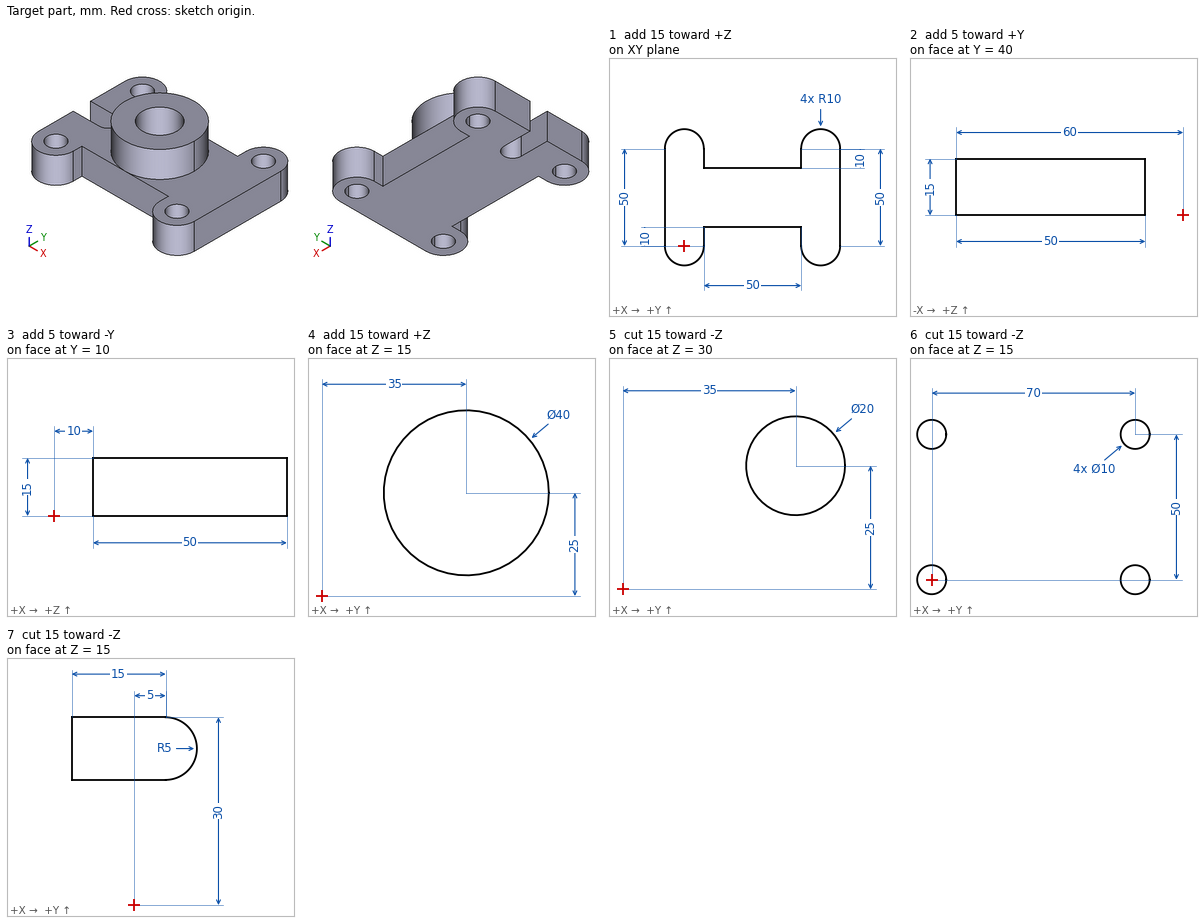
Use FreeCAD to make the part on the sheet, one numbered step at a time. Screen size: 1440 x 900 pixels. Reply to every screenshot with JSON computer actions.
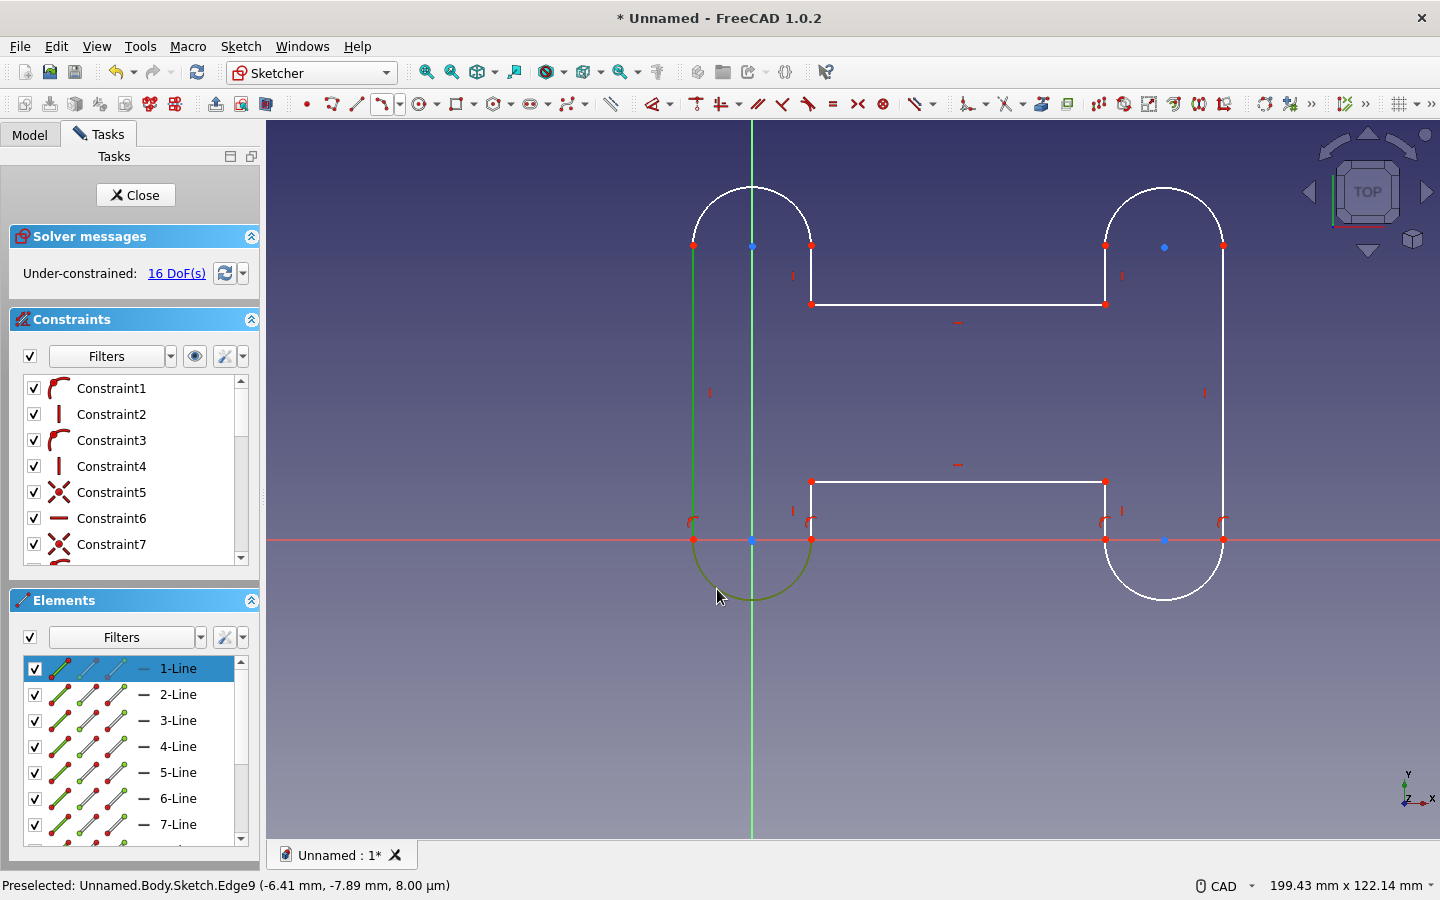
{"action": "key", "text": "t"}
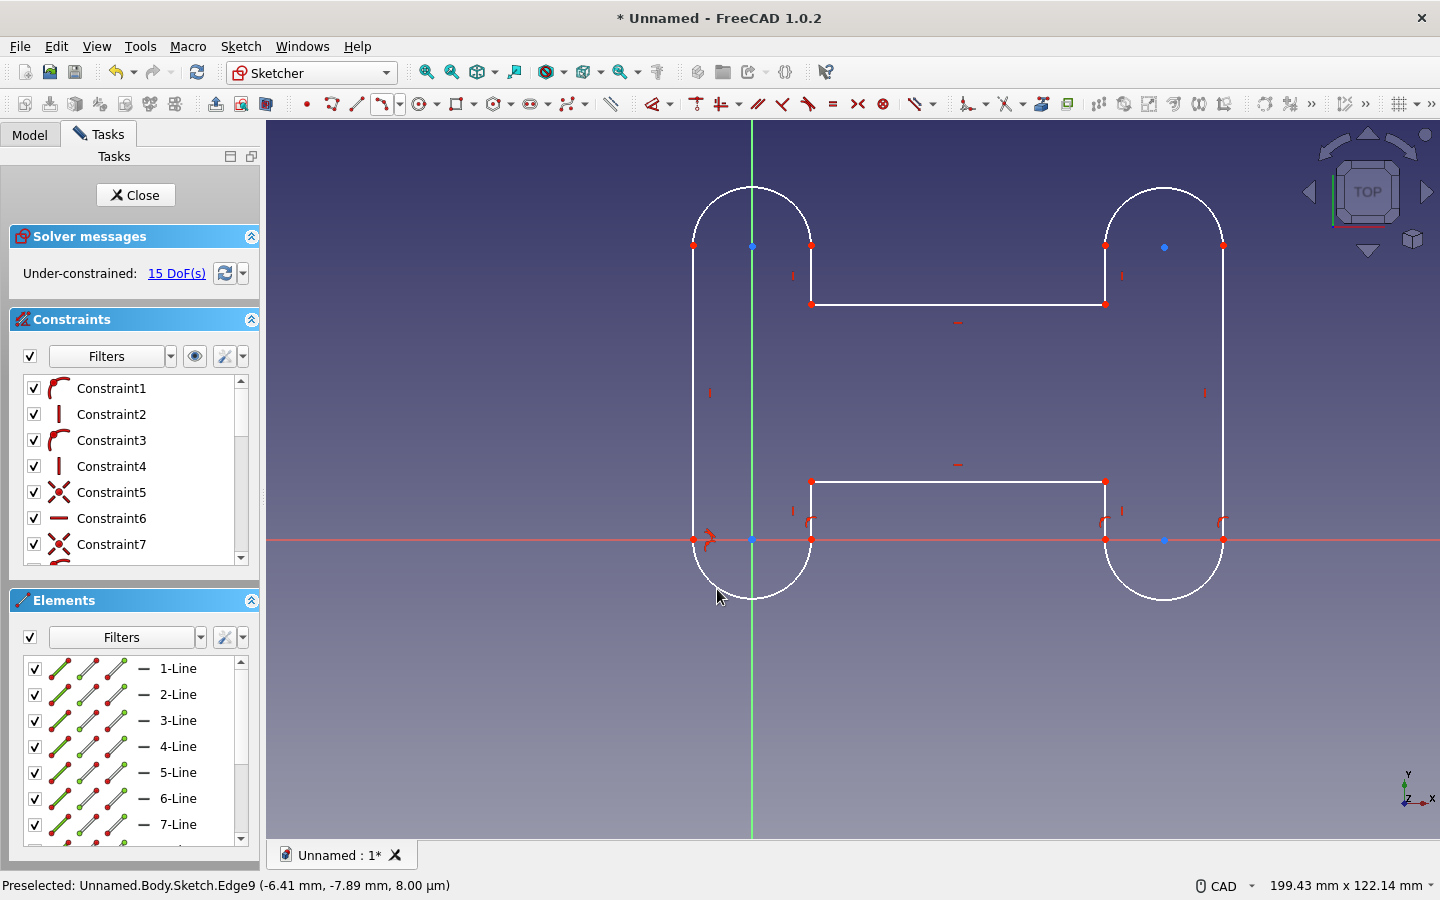
{"action": "left_click", "coordinate": [693, 334]}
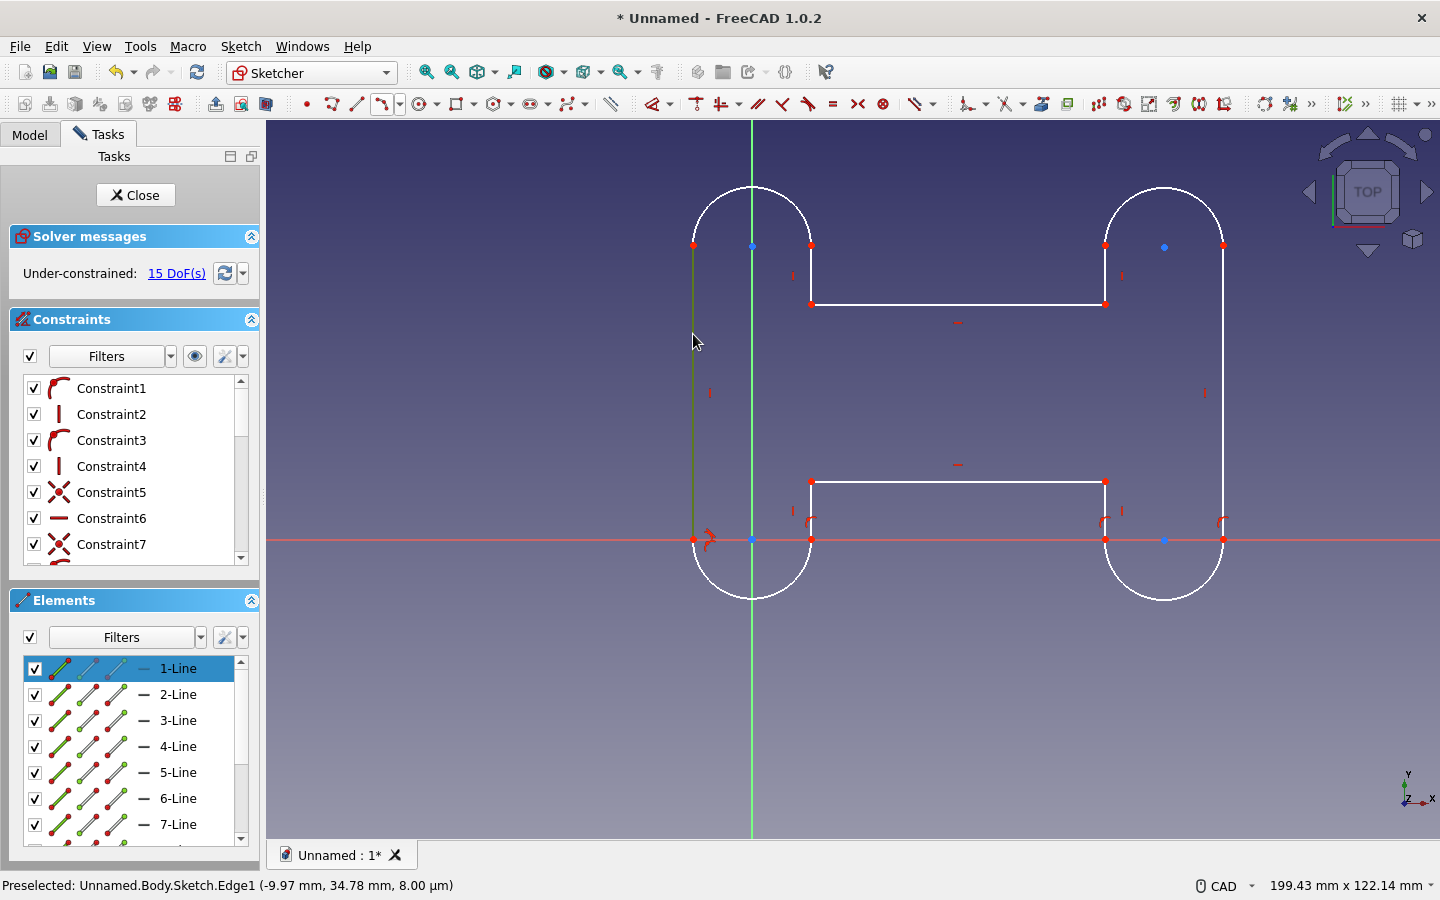
{"action": "left_click", "coordinate": [787, 198]}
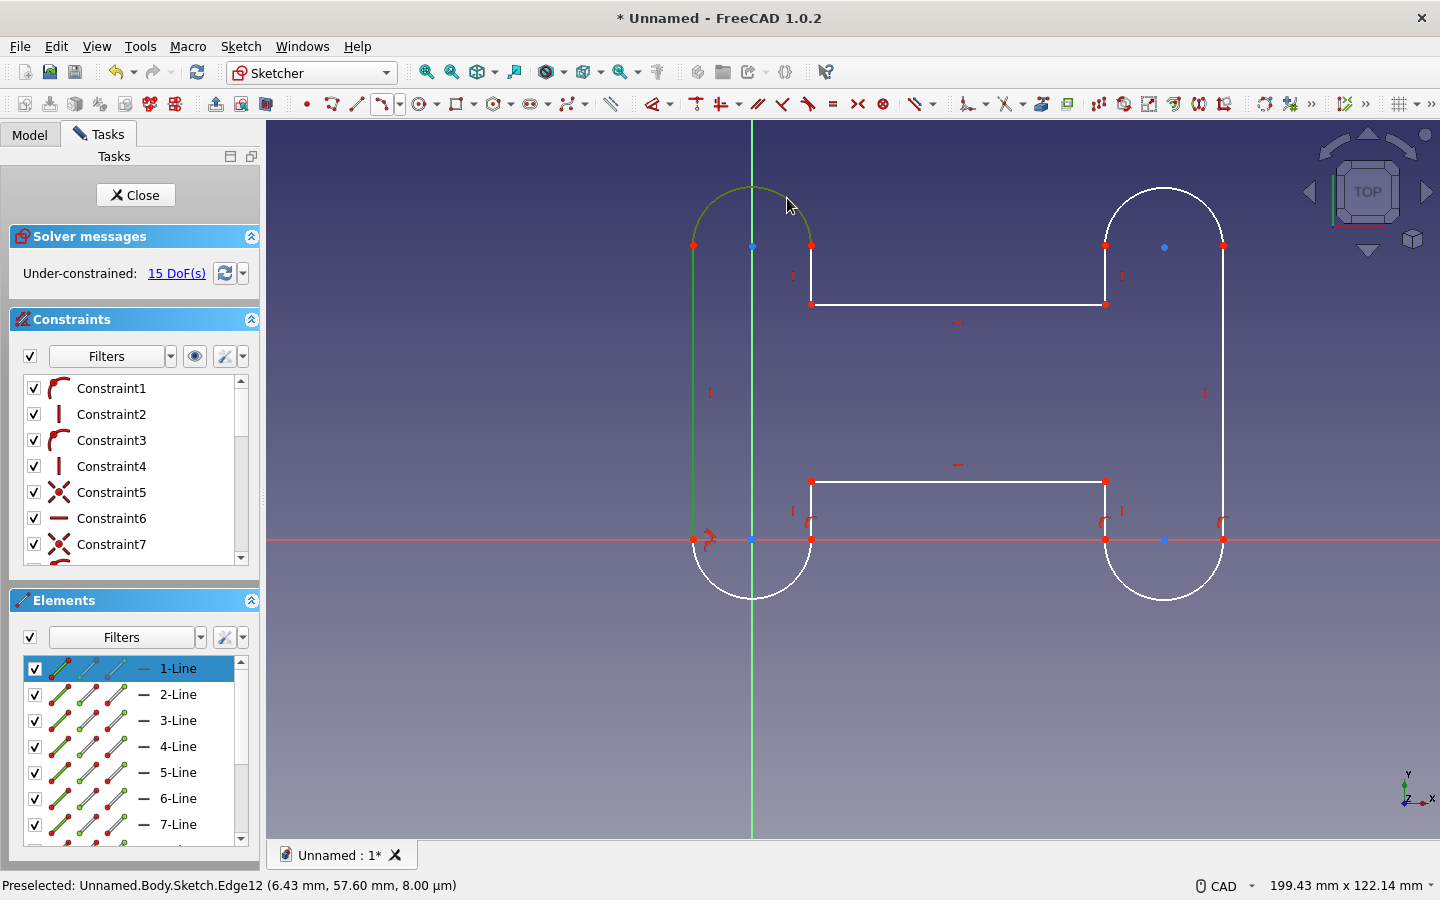
{"action": "left_click", "coordinate": [808, 104]}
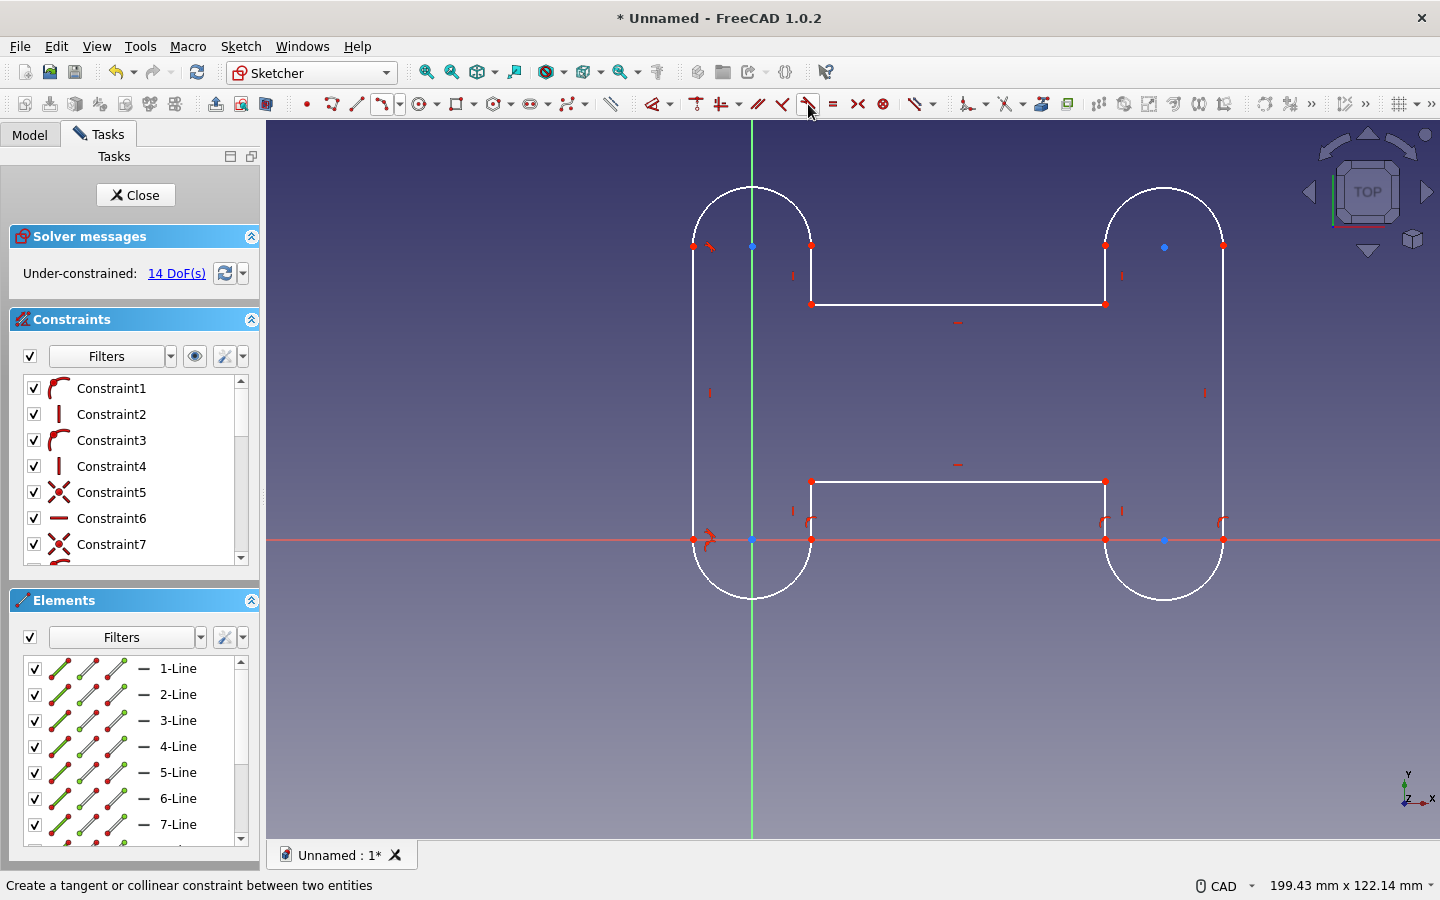
{"action": "left_click", "coordinate": [1105, 499]}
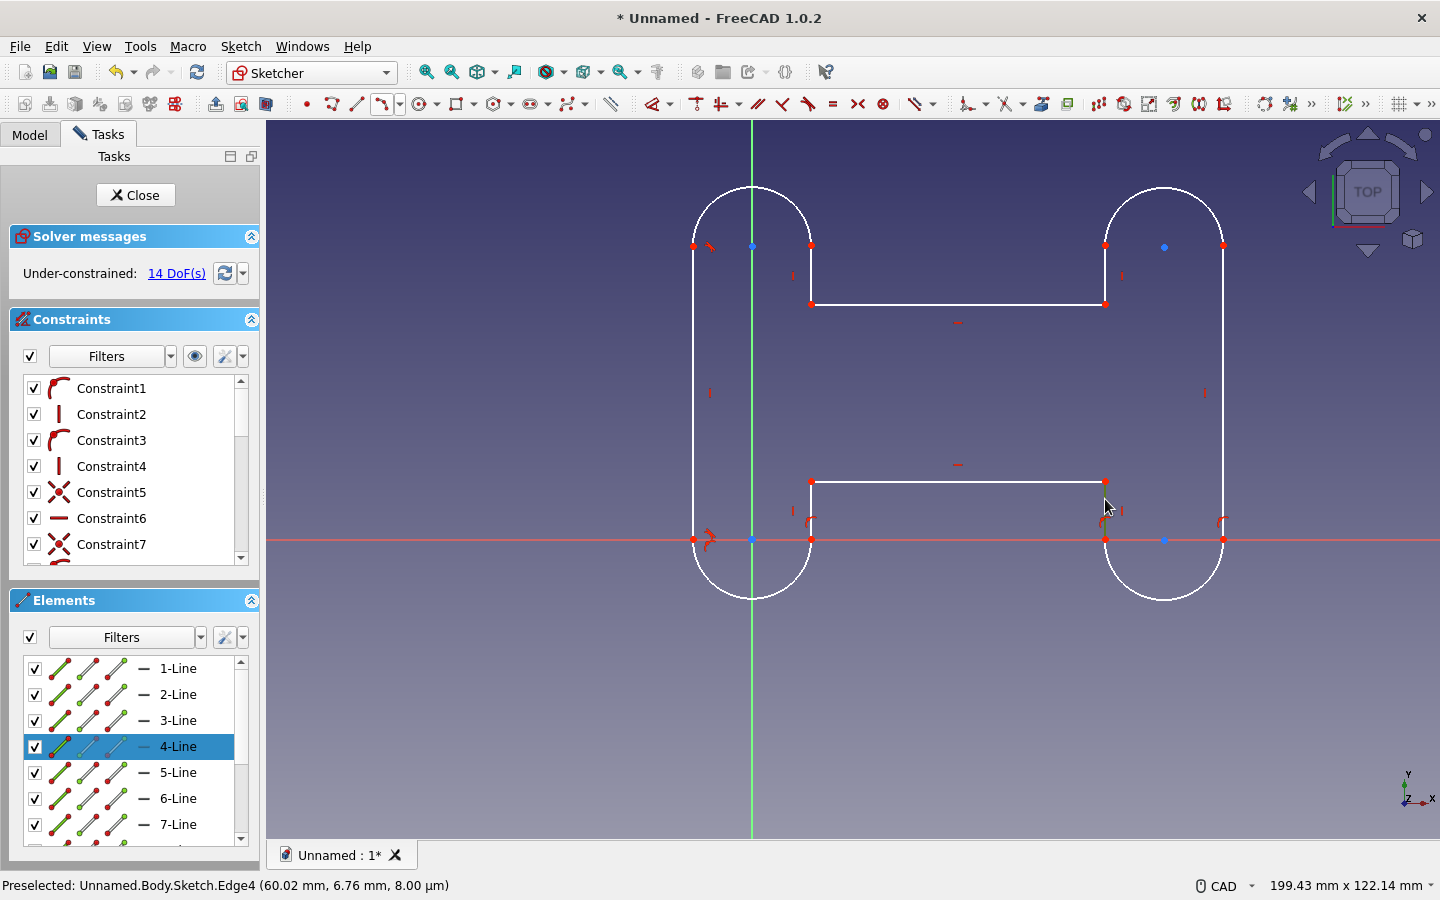
{"action": "left_click", "coordinate": [1129, 588]}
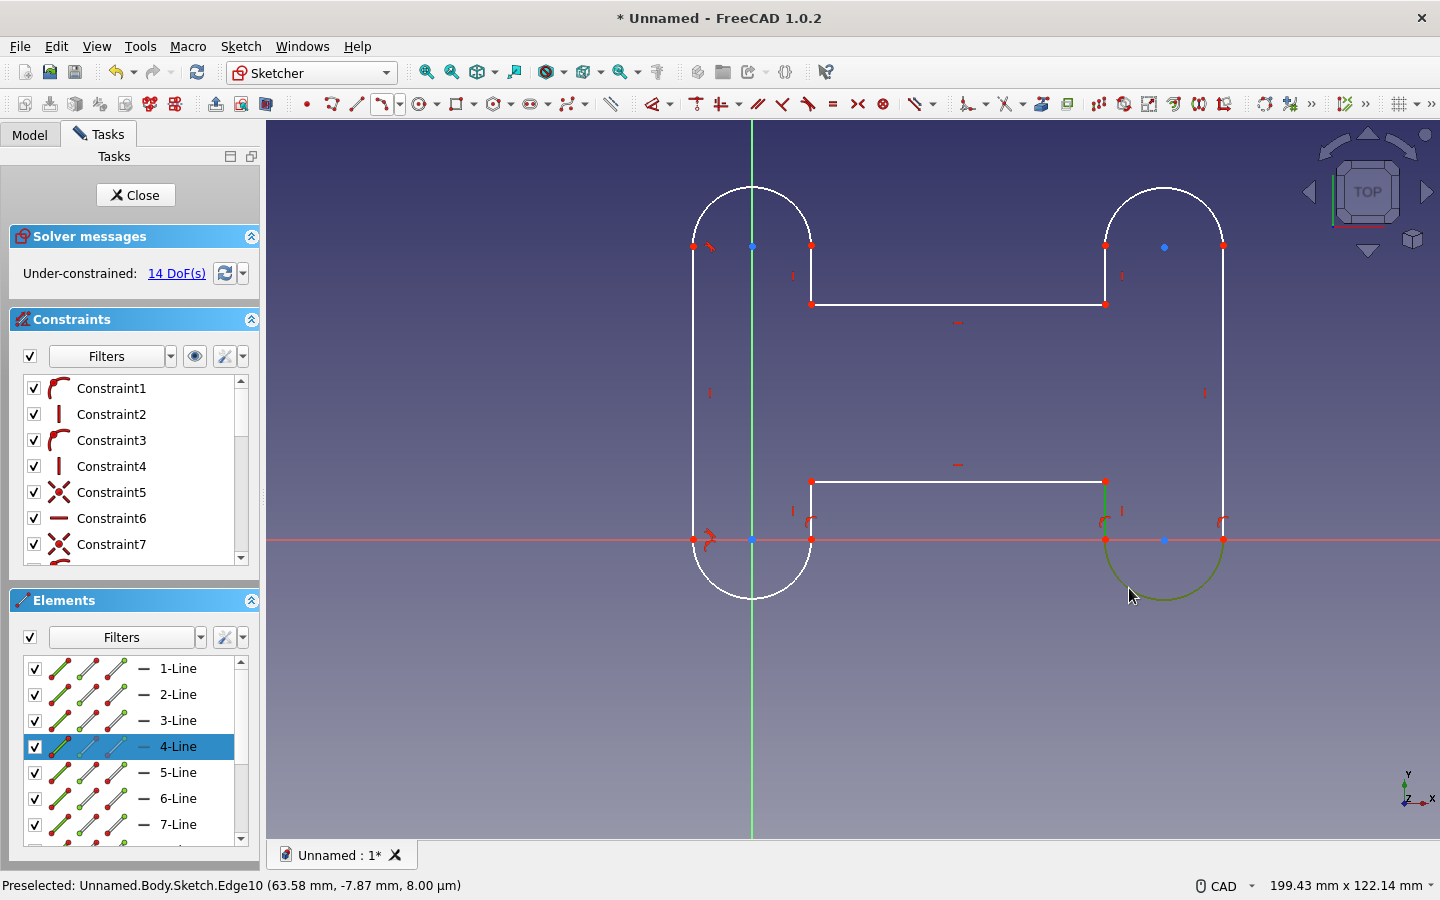
{"action": "left_click", "coordinate": [808, 104]}